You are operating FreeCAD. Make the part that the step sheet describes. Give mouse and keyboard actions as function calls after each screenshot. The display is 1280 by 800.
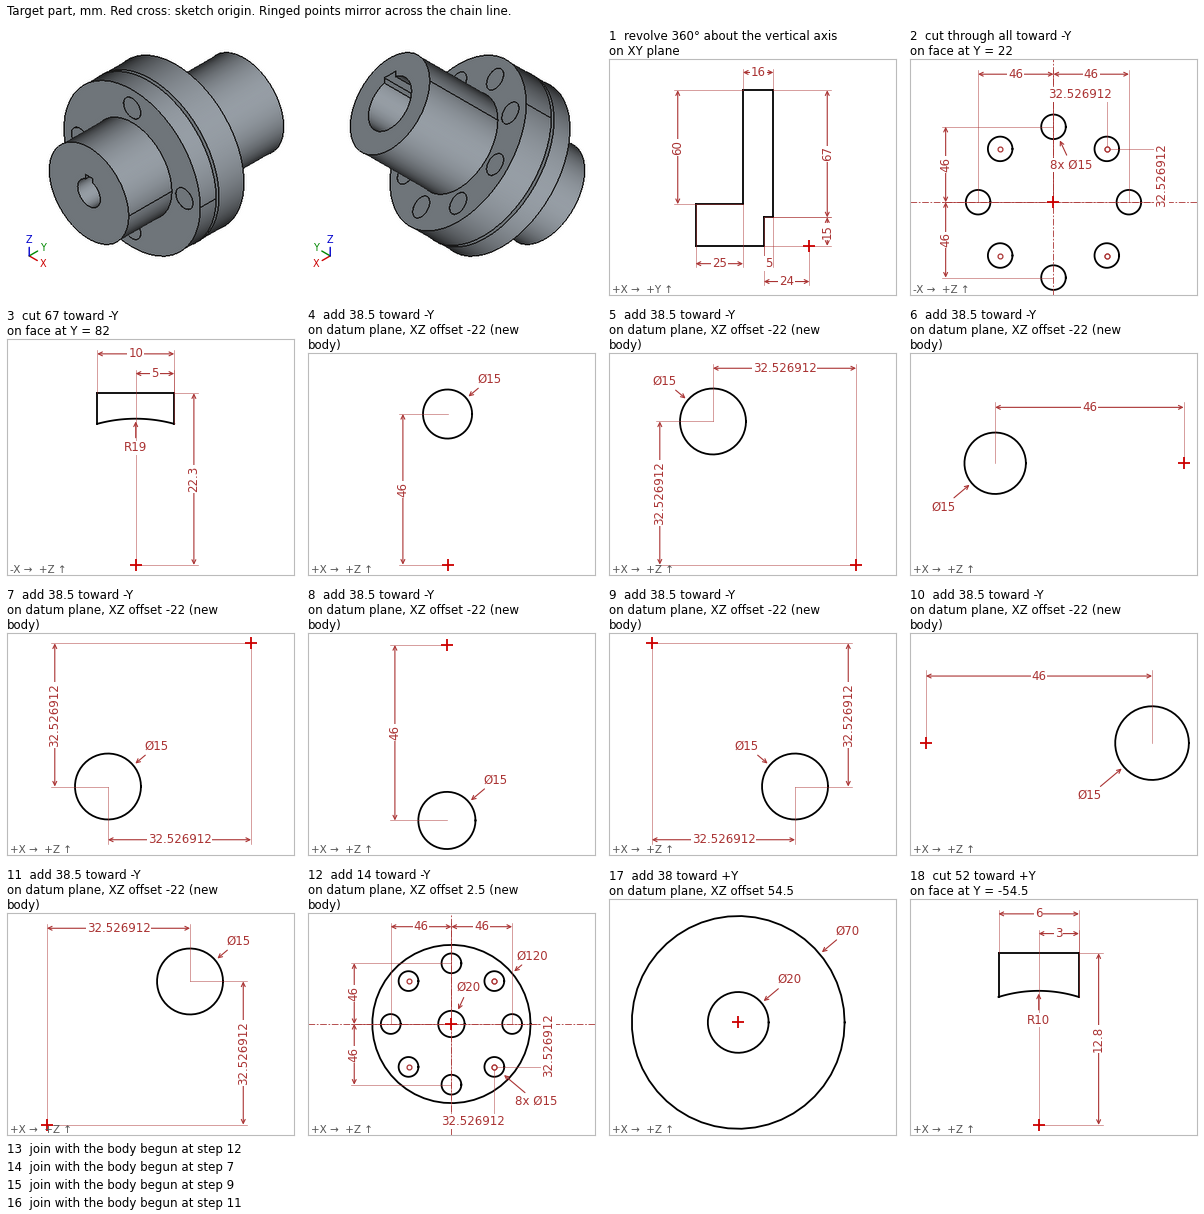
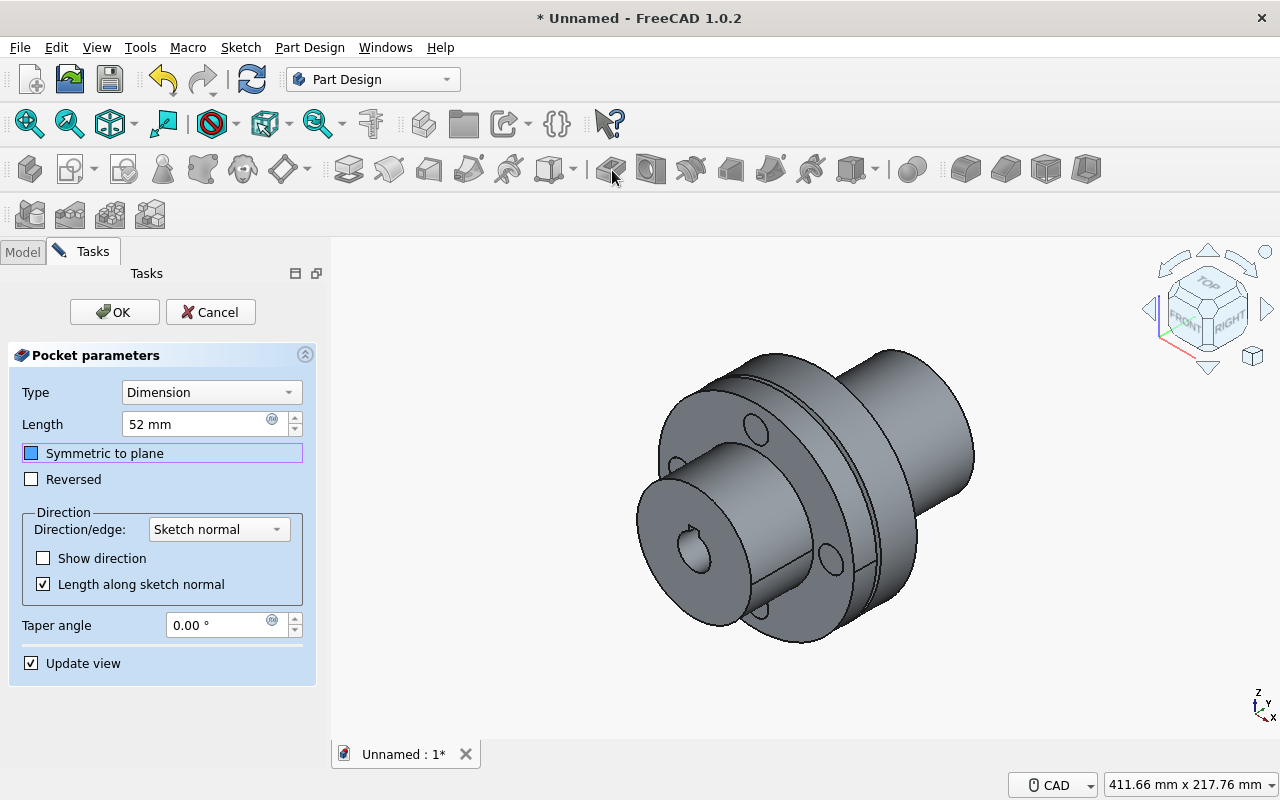
click(115, 312)